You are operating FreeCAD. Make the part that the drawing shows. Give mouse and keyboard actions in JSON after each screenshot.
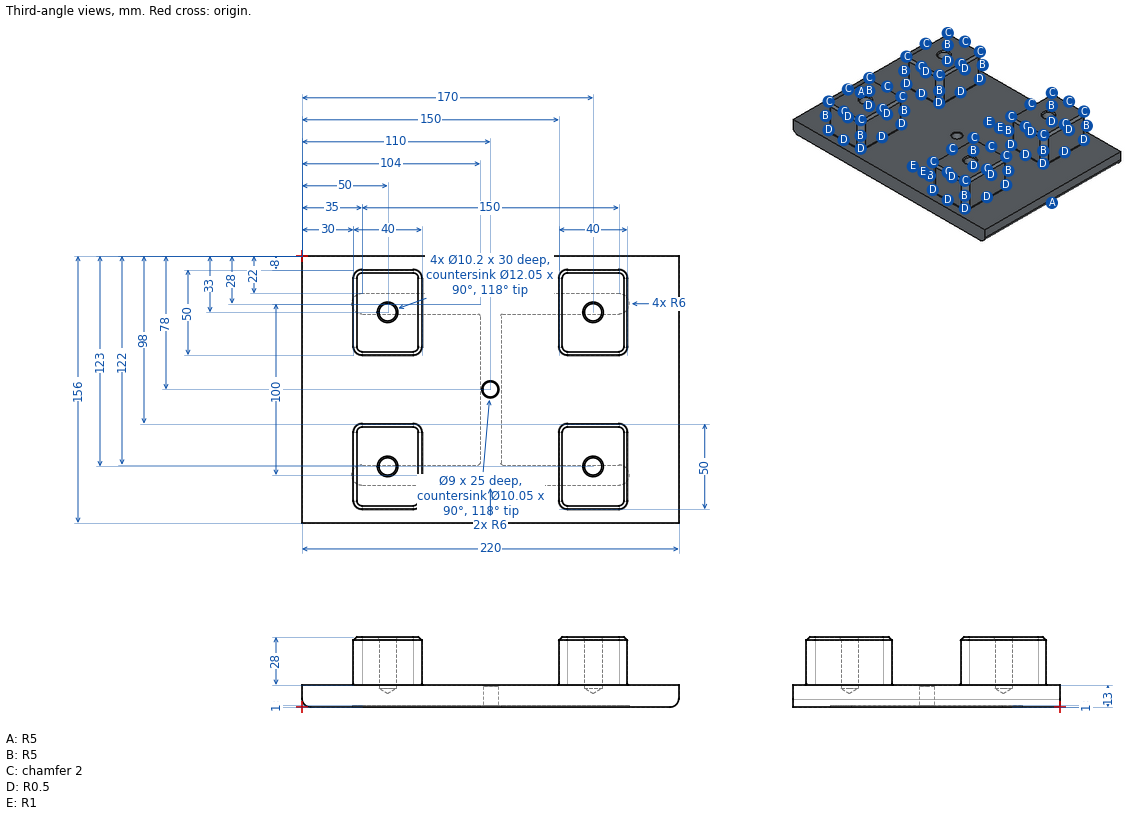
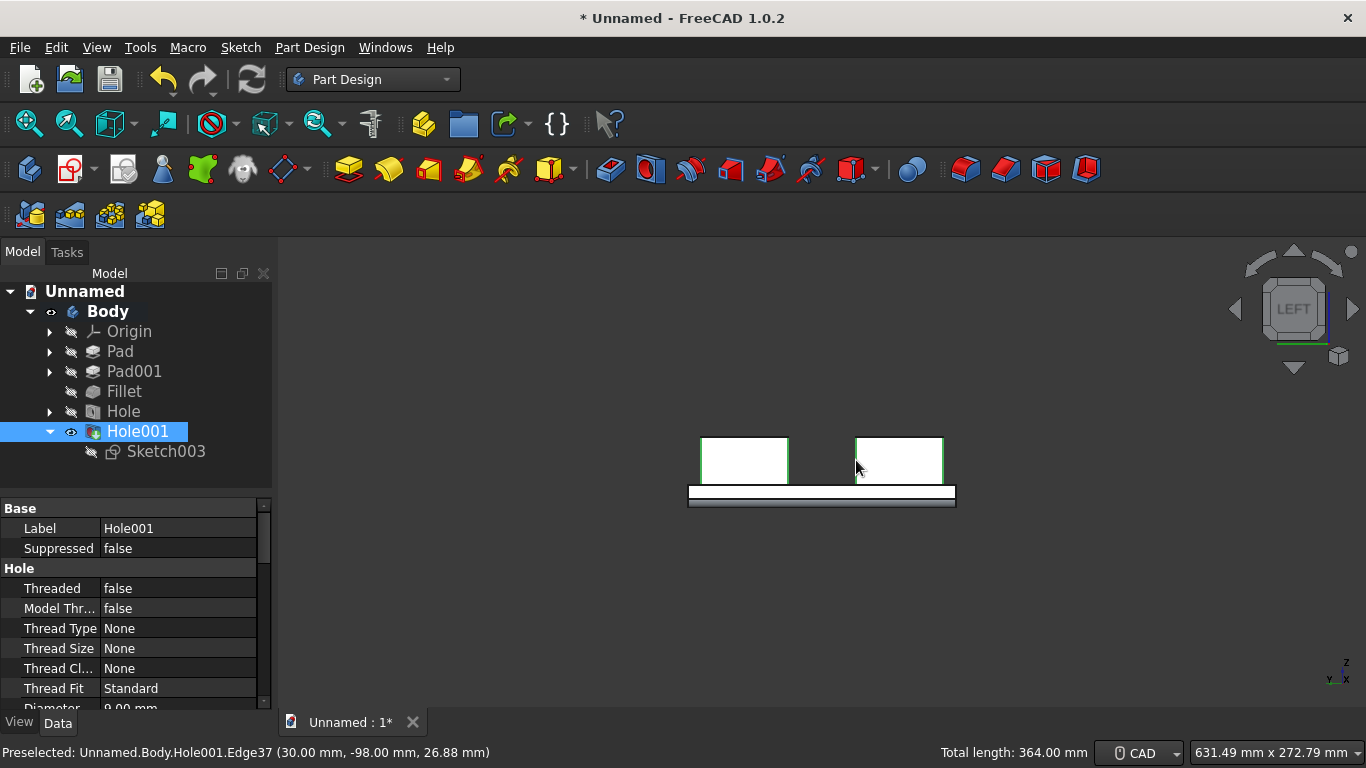
{"action": "key", "text": "v 3"}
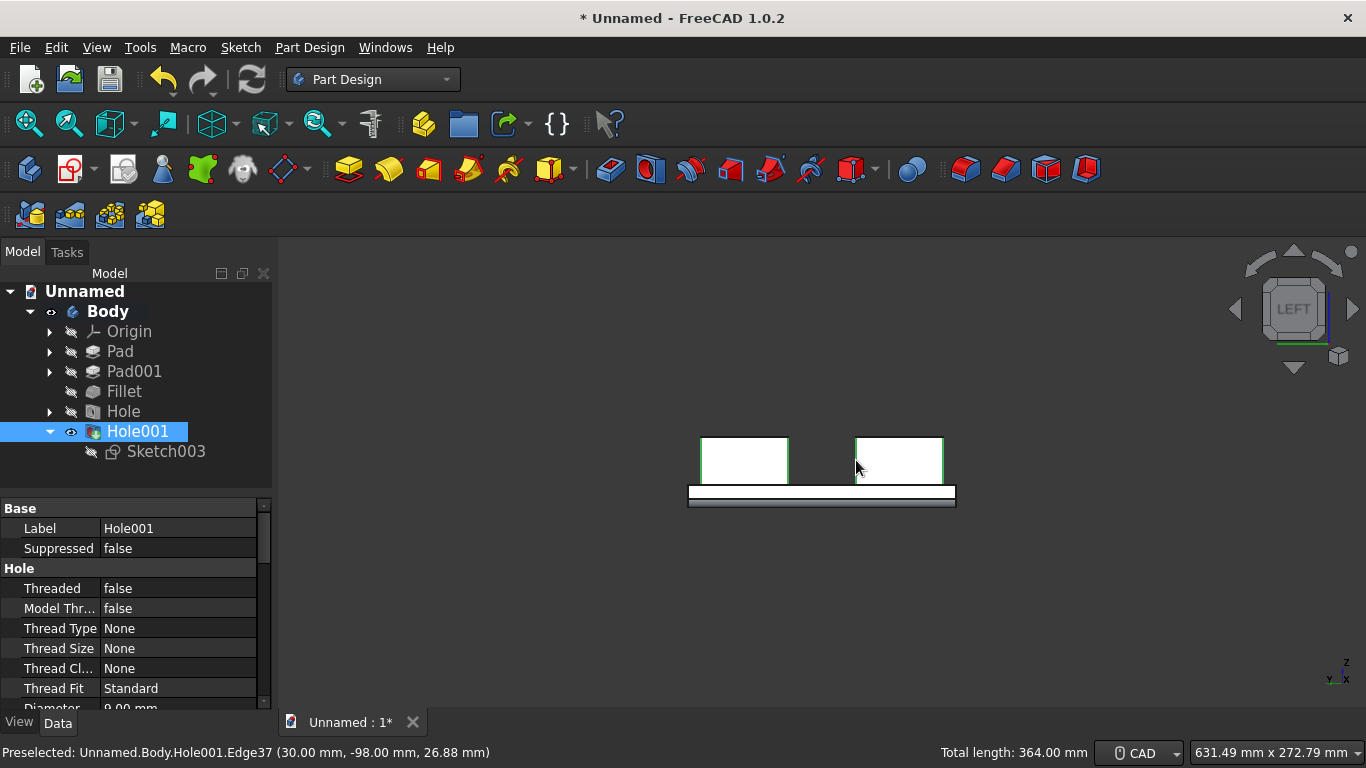
{"action": "key", "text": "0"}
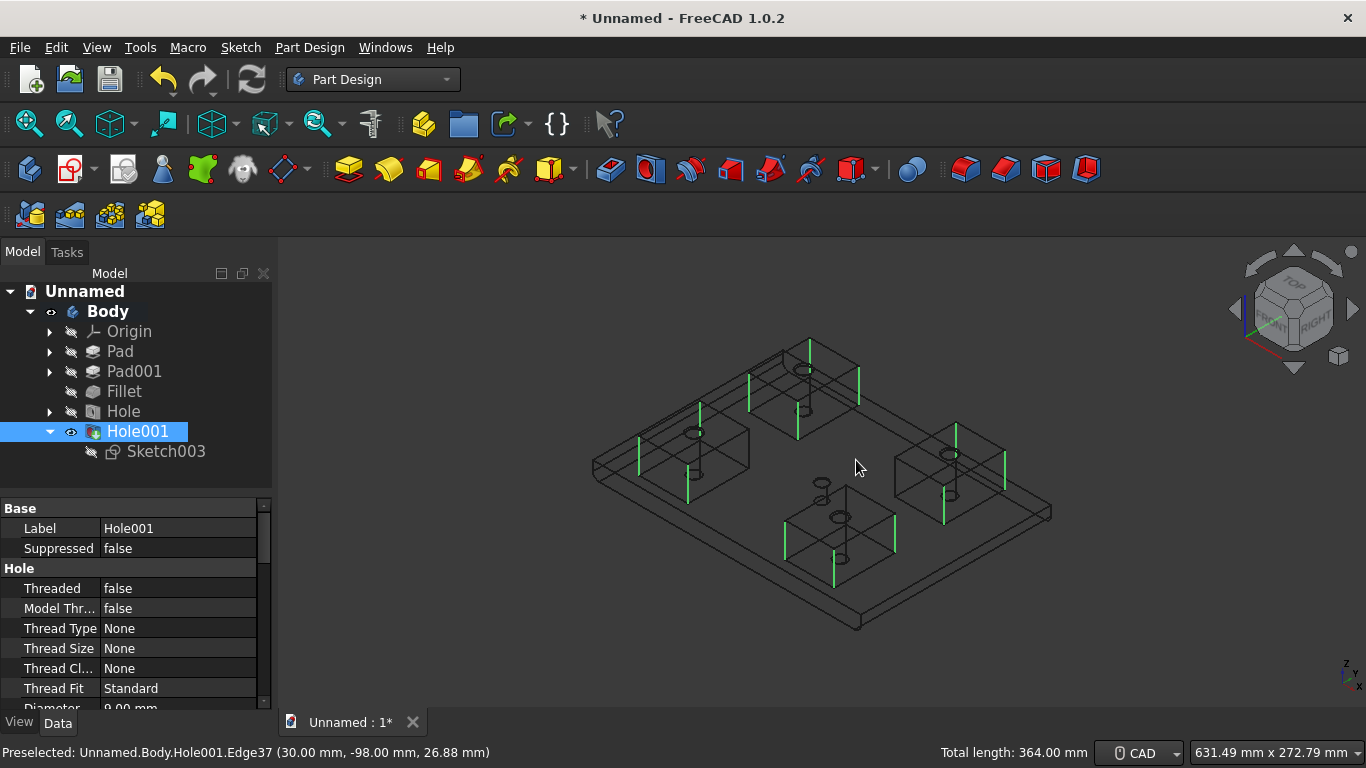
{"action": "left_click", "coordinate": [895, 476], "text": "ctrl"}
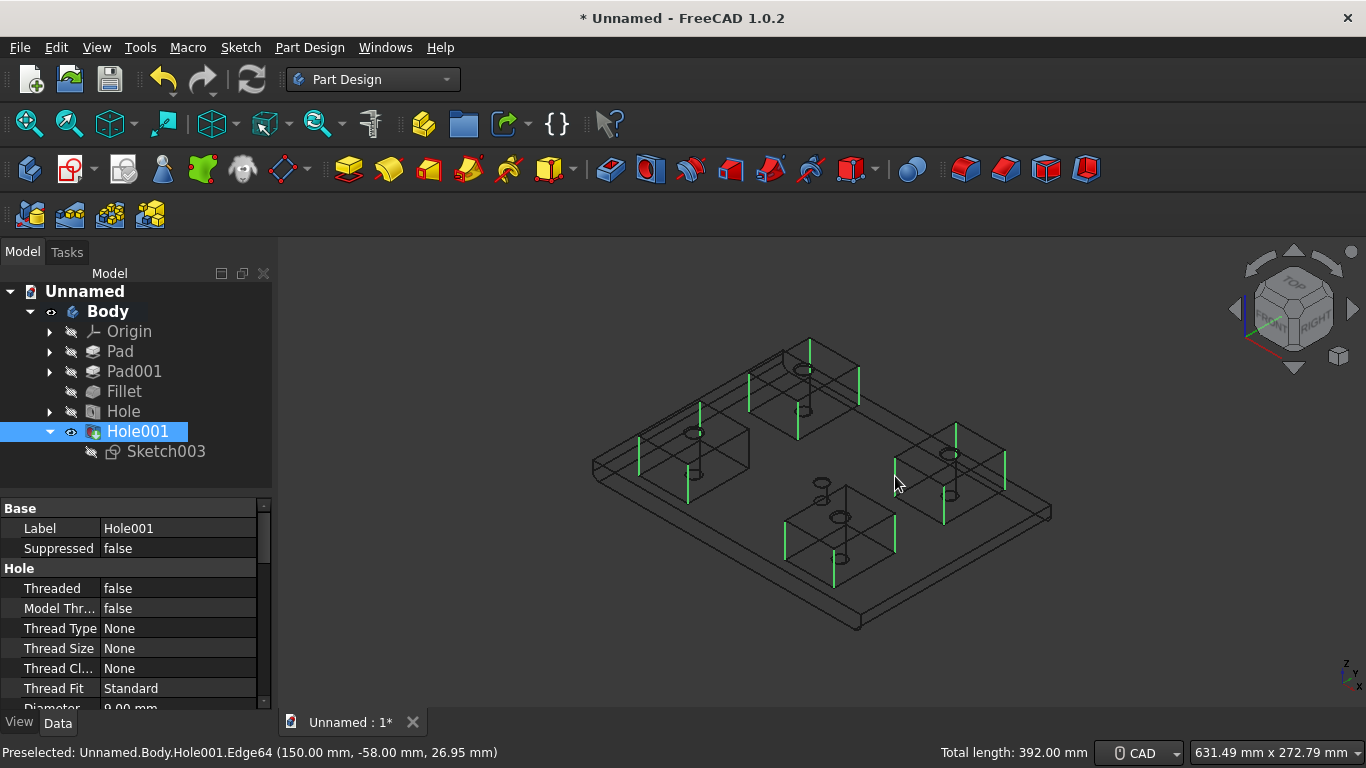
{"action": "left_click", "coordinate": [846, 504], "text": "ctrl"}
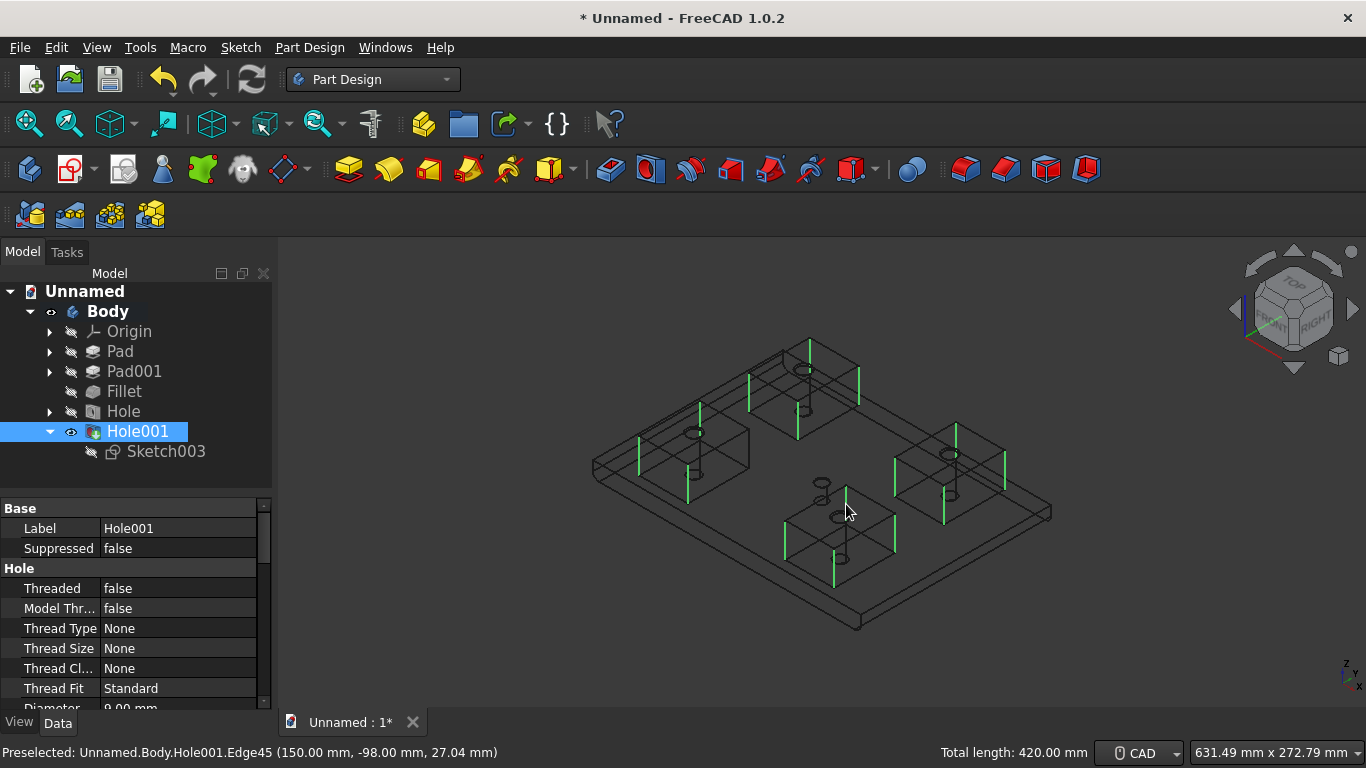
{"action": "left_click", "coordinate": [749, 448], "text": "ctrl"}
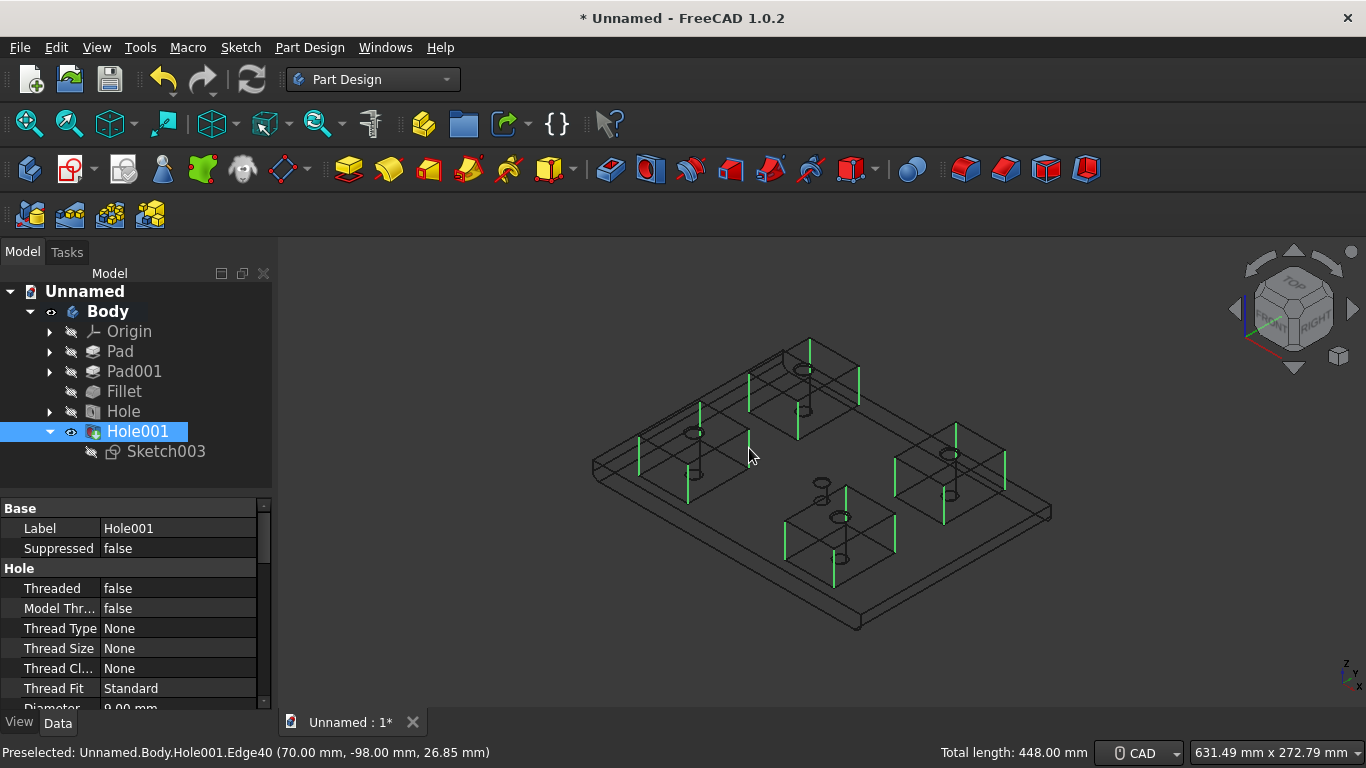
{"action": "key", "text": "v 1"}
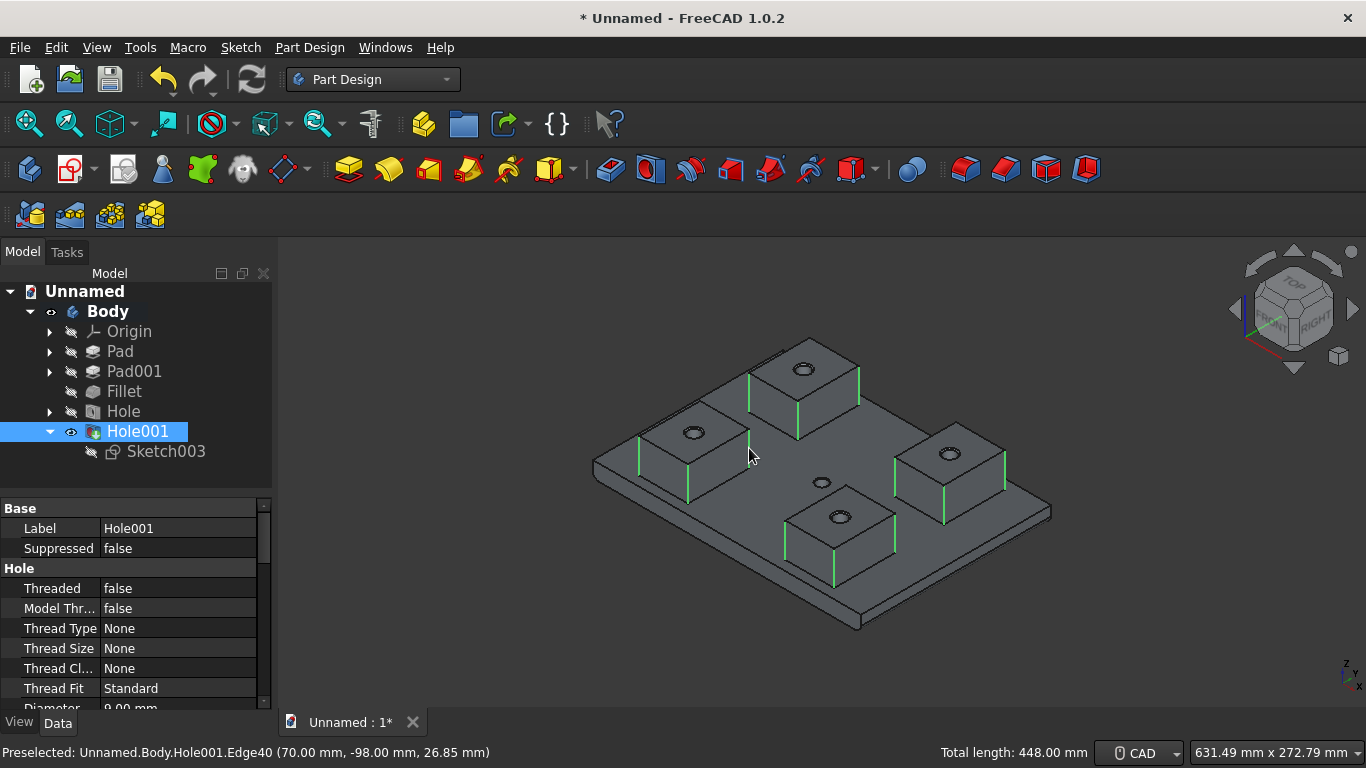
{"action": "left_click", "coordinate": [966, 170]}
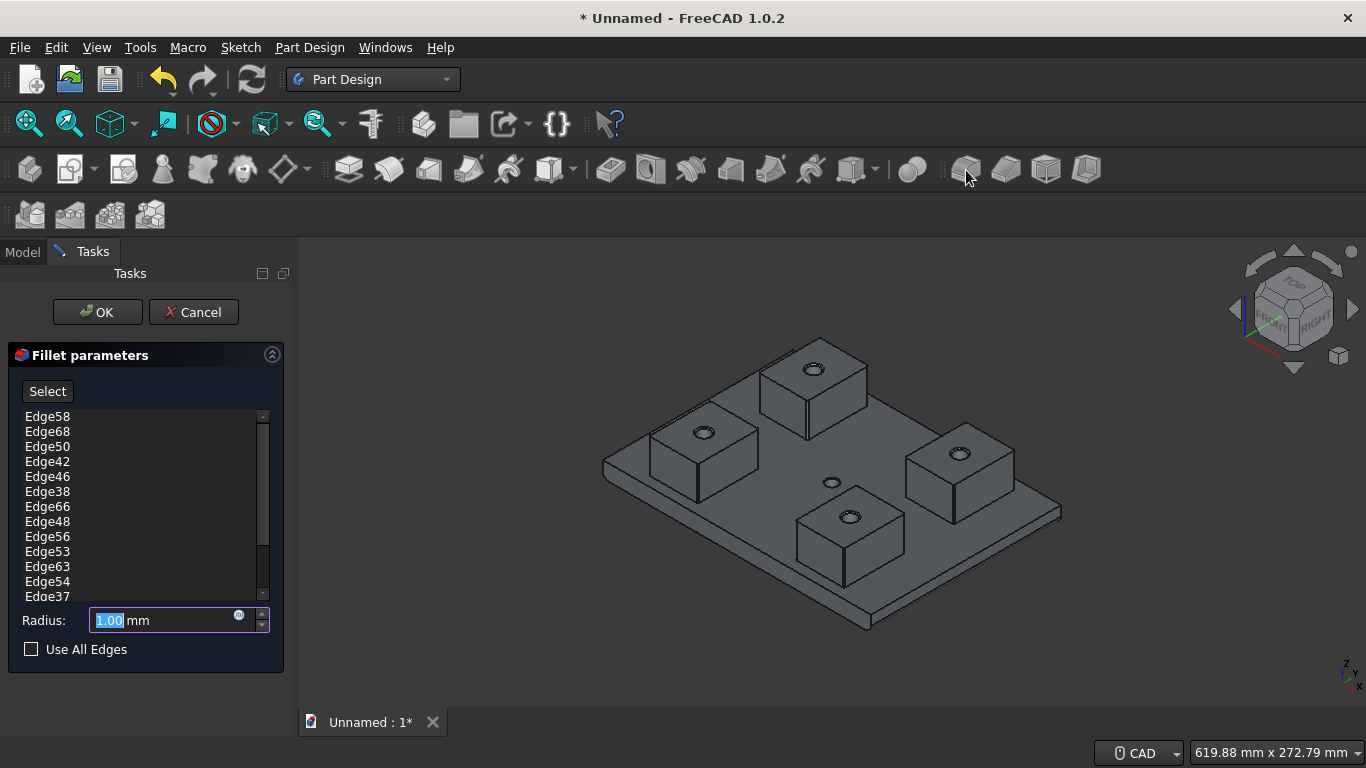
{"action": "type", "text": "5"}
{"action": "key", "text": "Tab"}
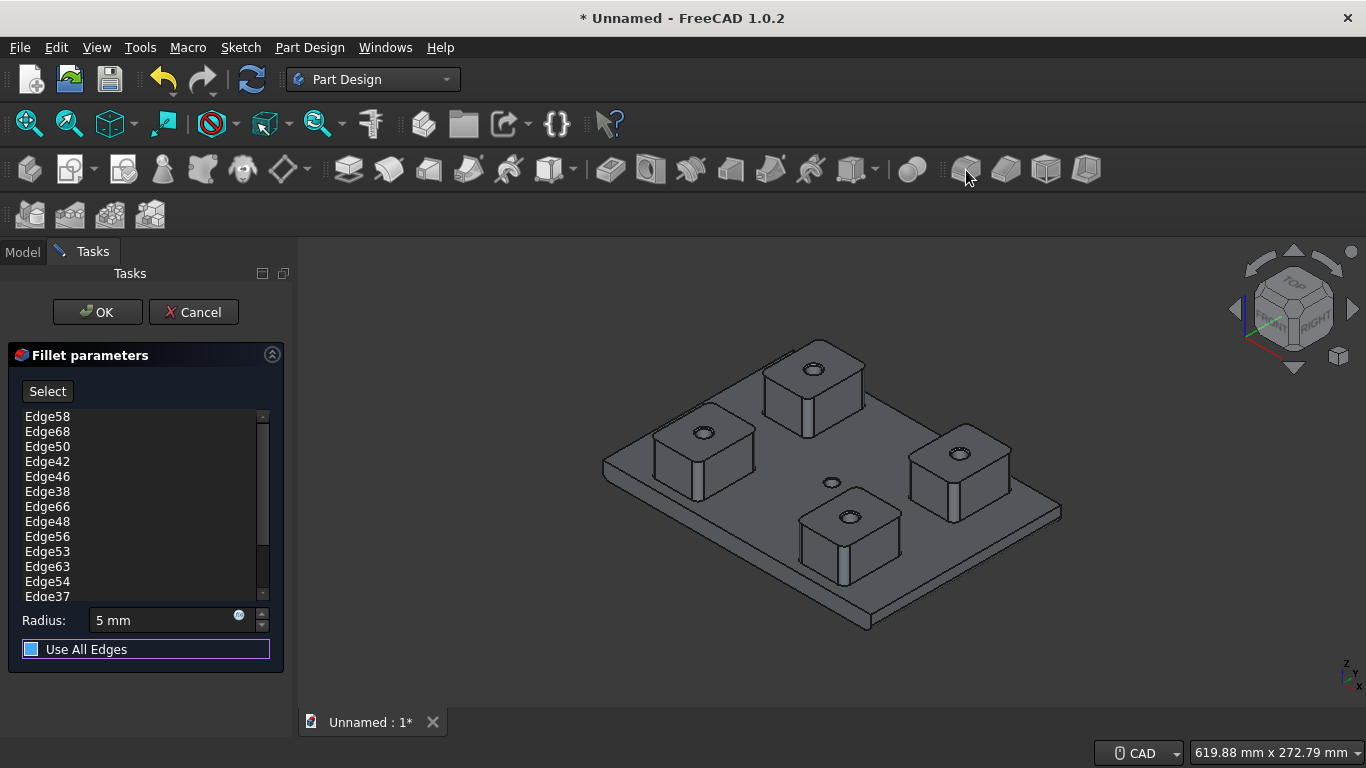
{"action": "left_click", "coordinate": [98, 312]}